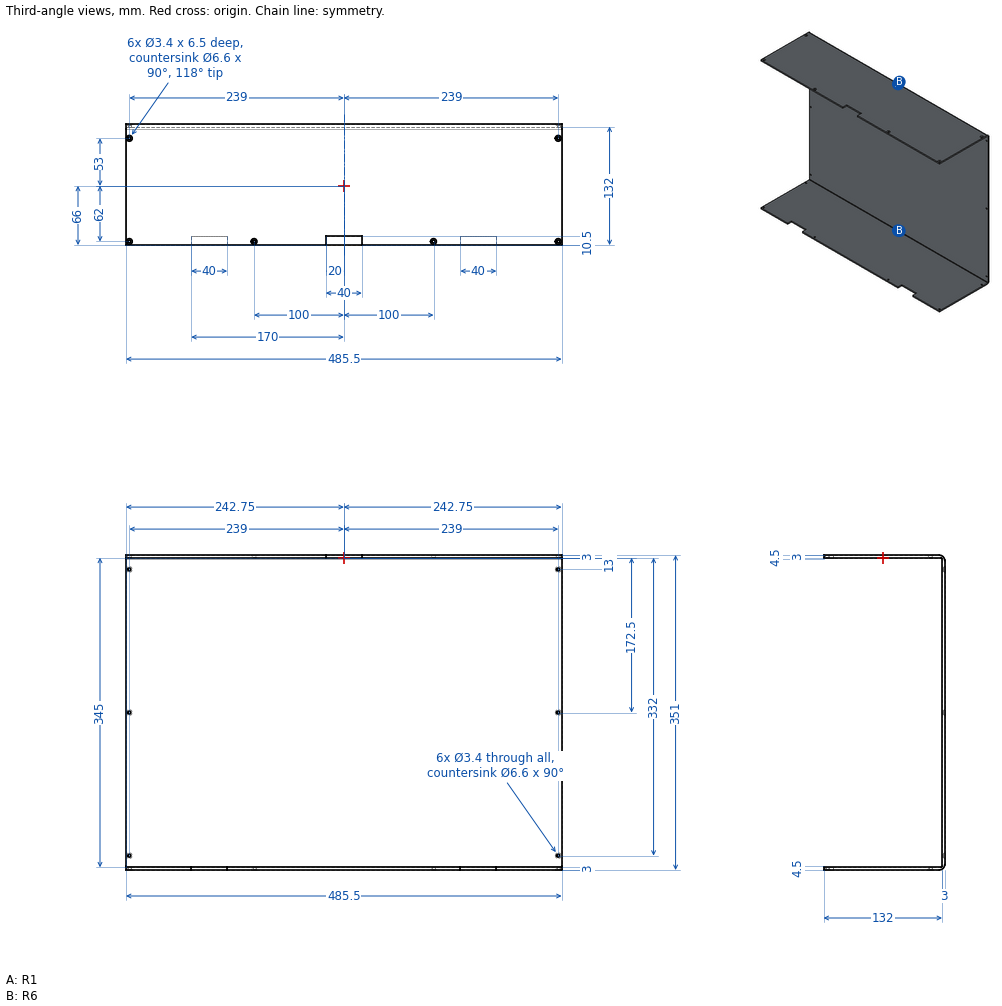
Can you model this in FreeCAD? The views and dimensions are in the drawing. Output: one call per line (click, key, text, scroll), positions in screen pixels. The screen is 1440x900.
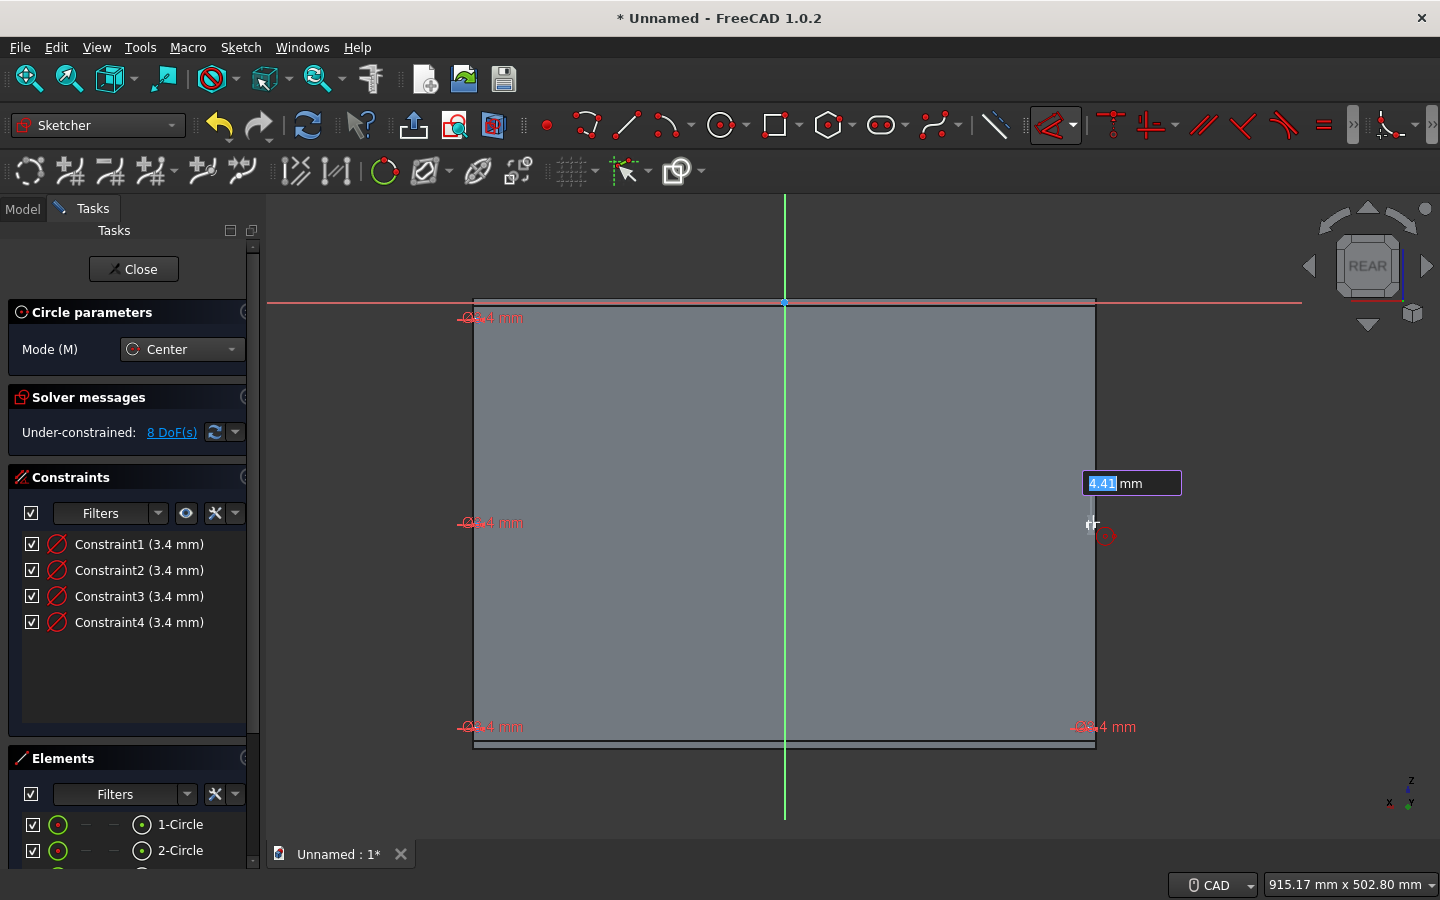
text(3.4)
key(Return)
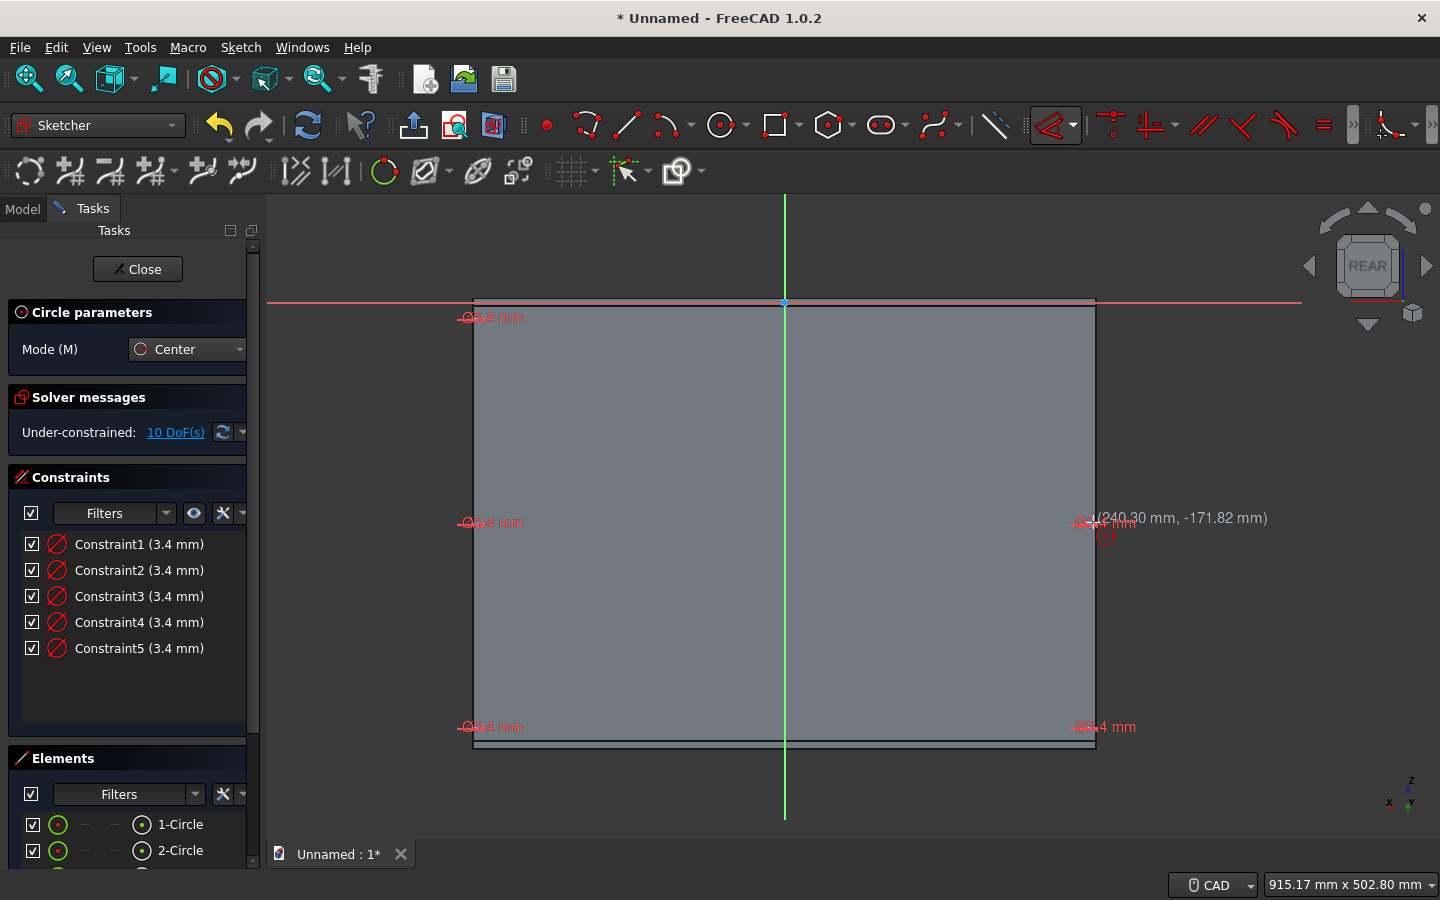
scroll(1091, 319, up, 12)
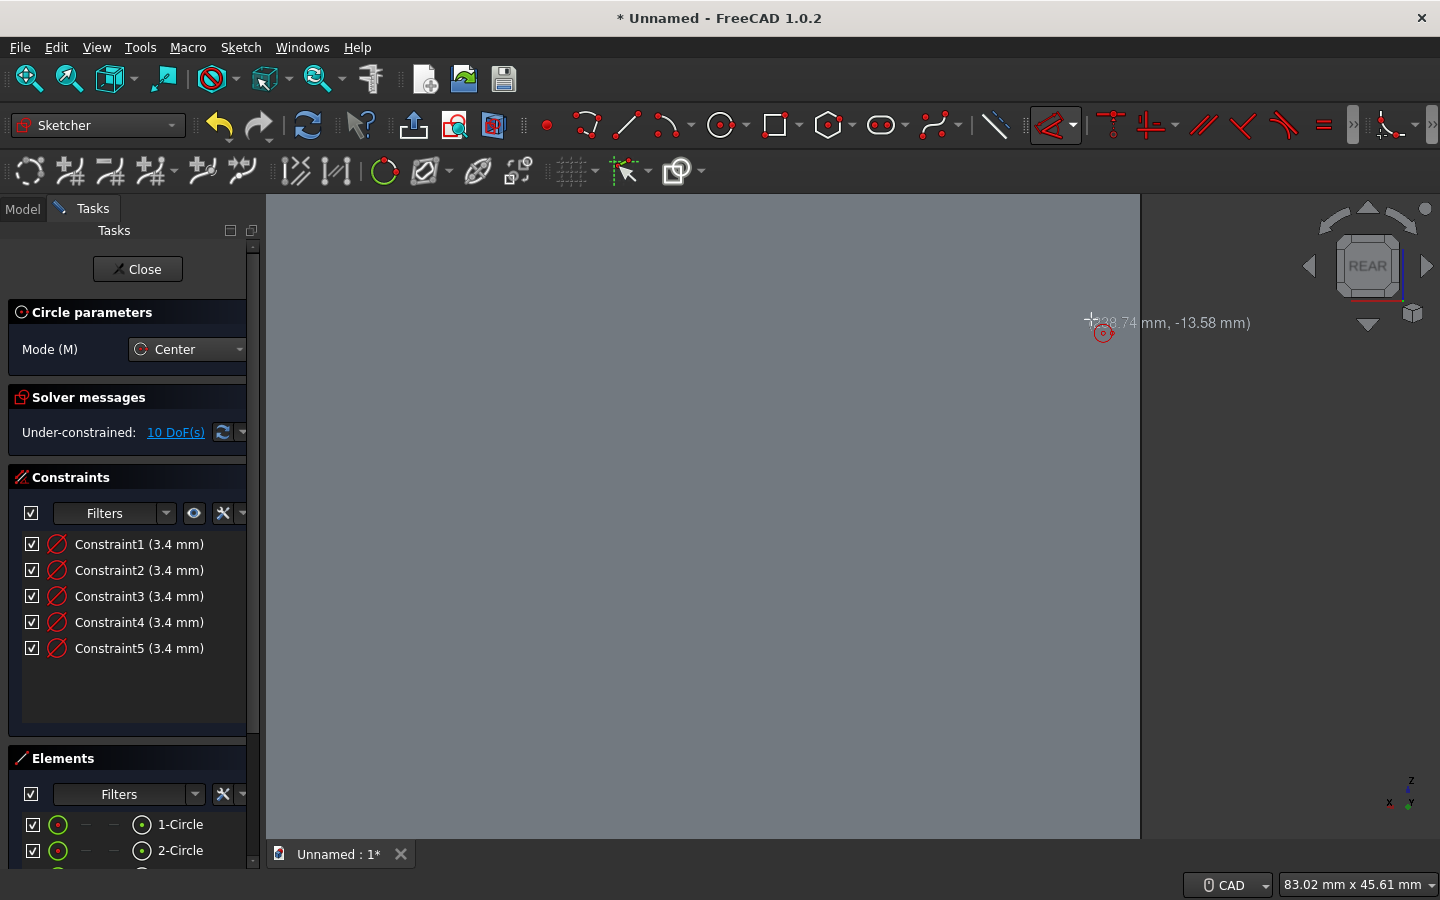
scroll(1091, 319, down, 12)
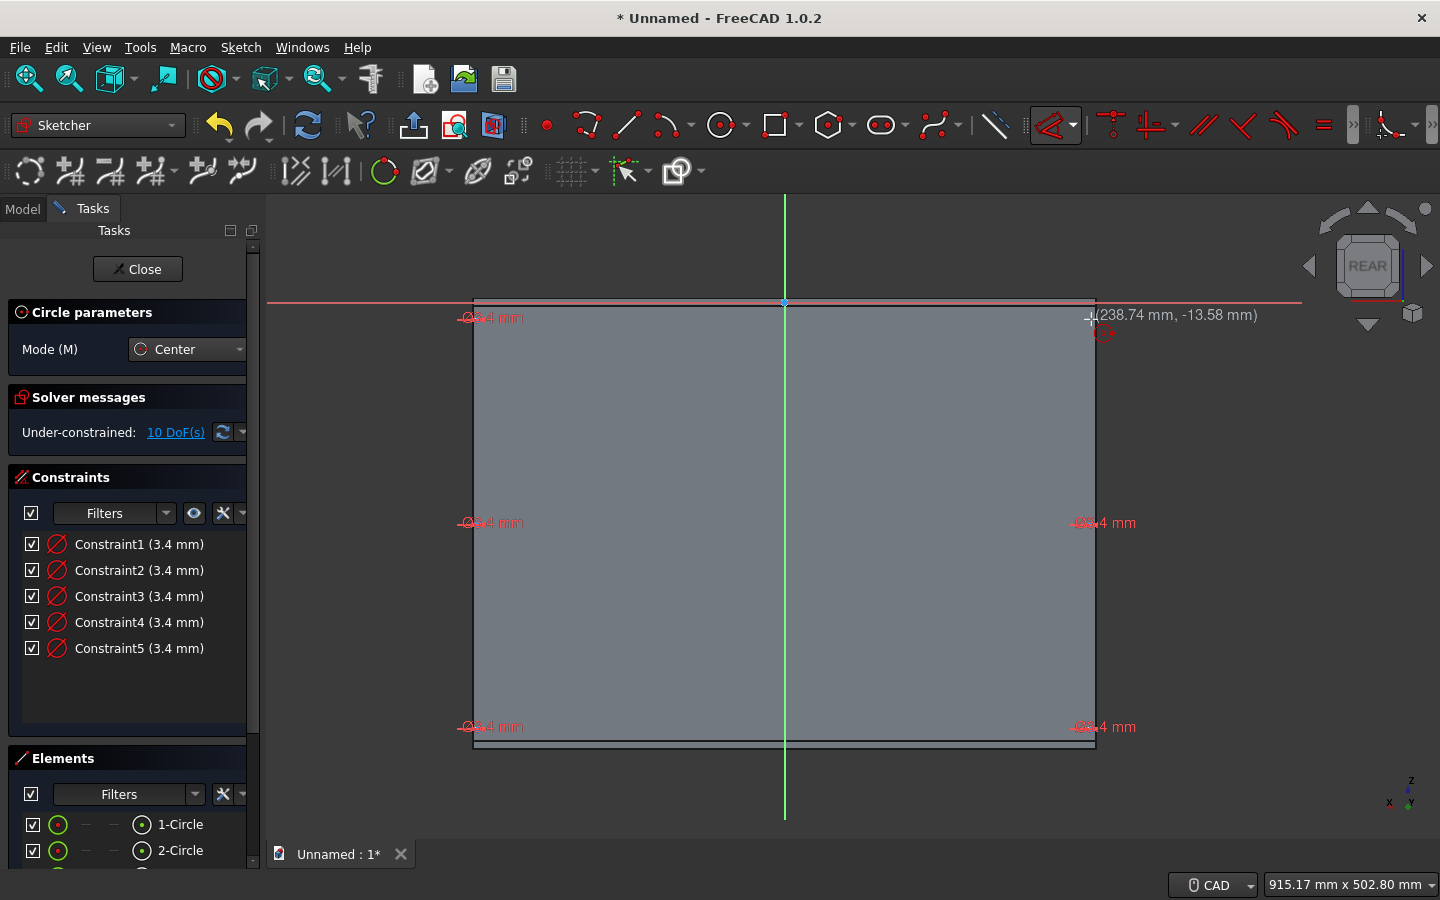
click(1091, 319)
move(1093, 318)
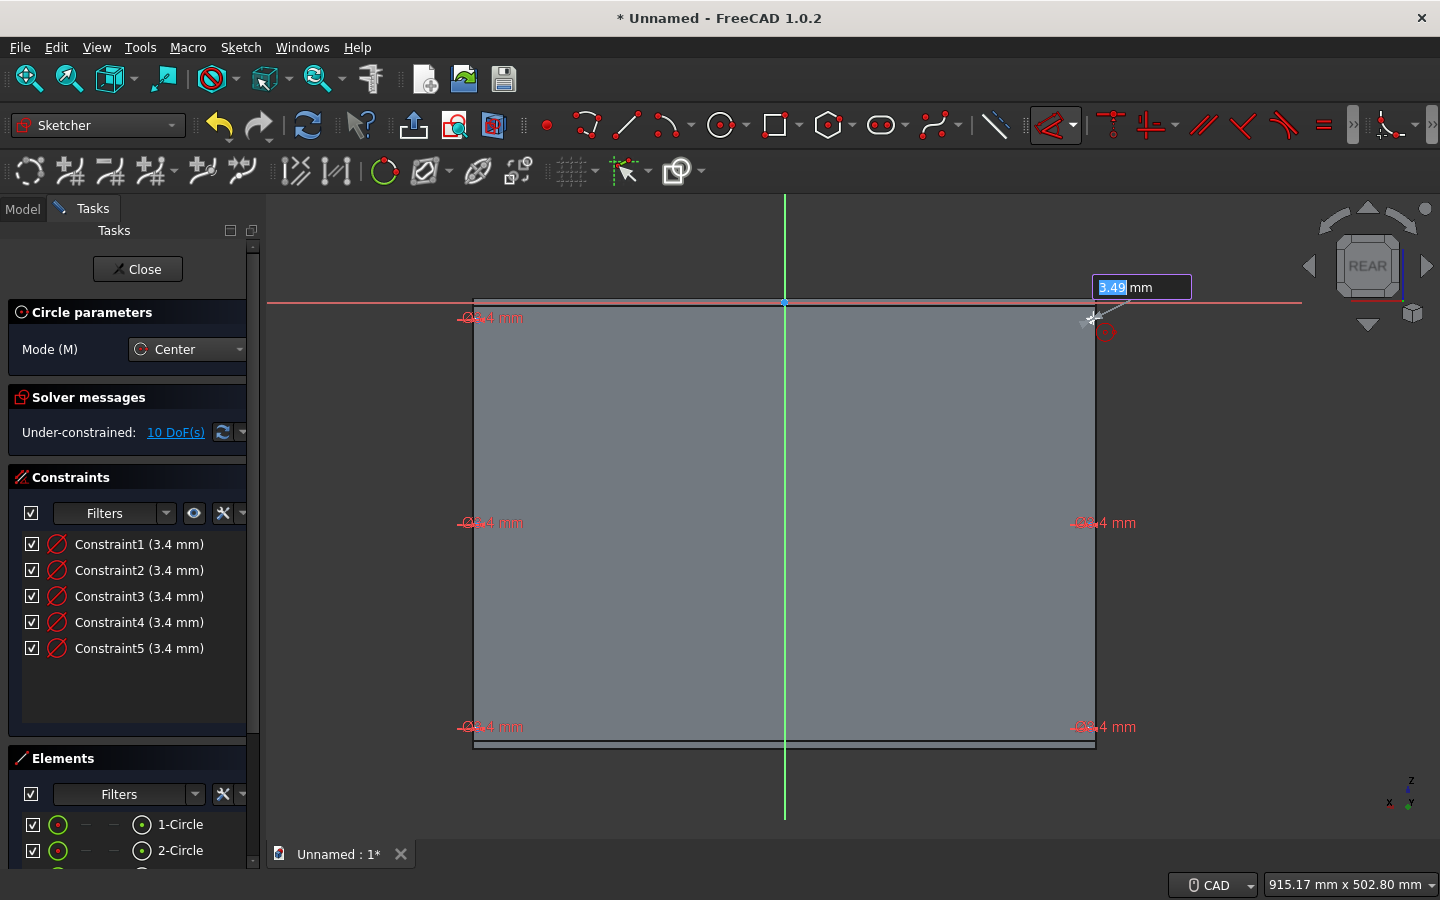
text(3.4)
key(Return)
key(Escape)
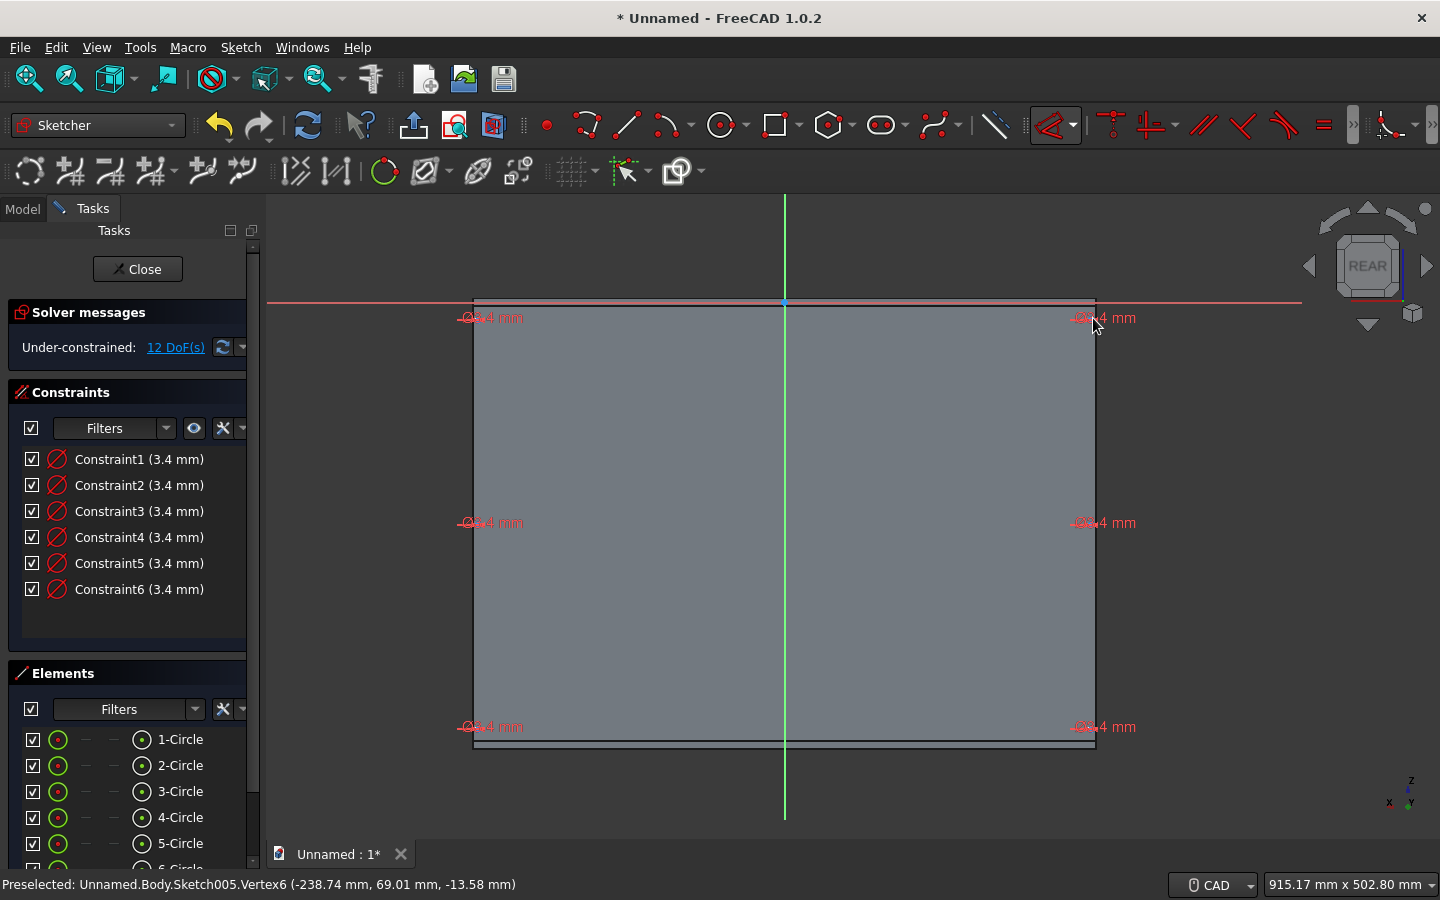
click(478, 729)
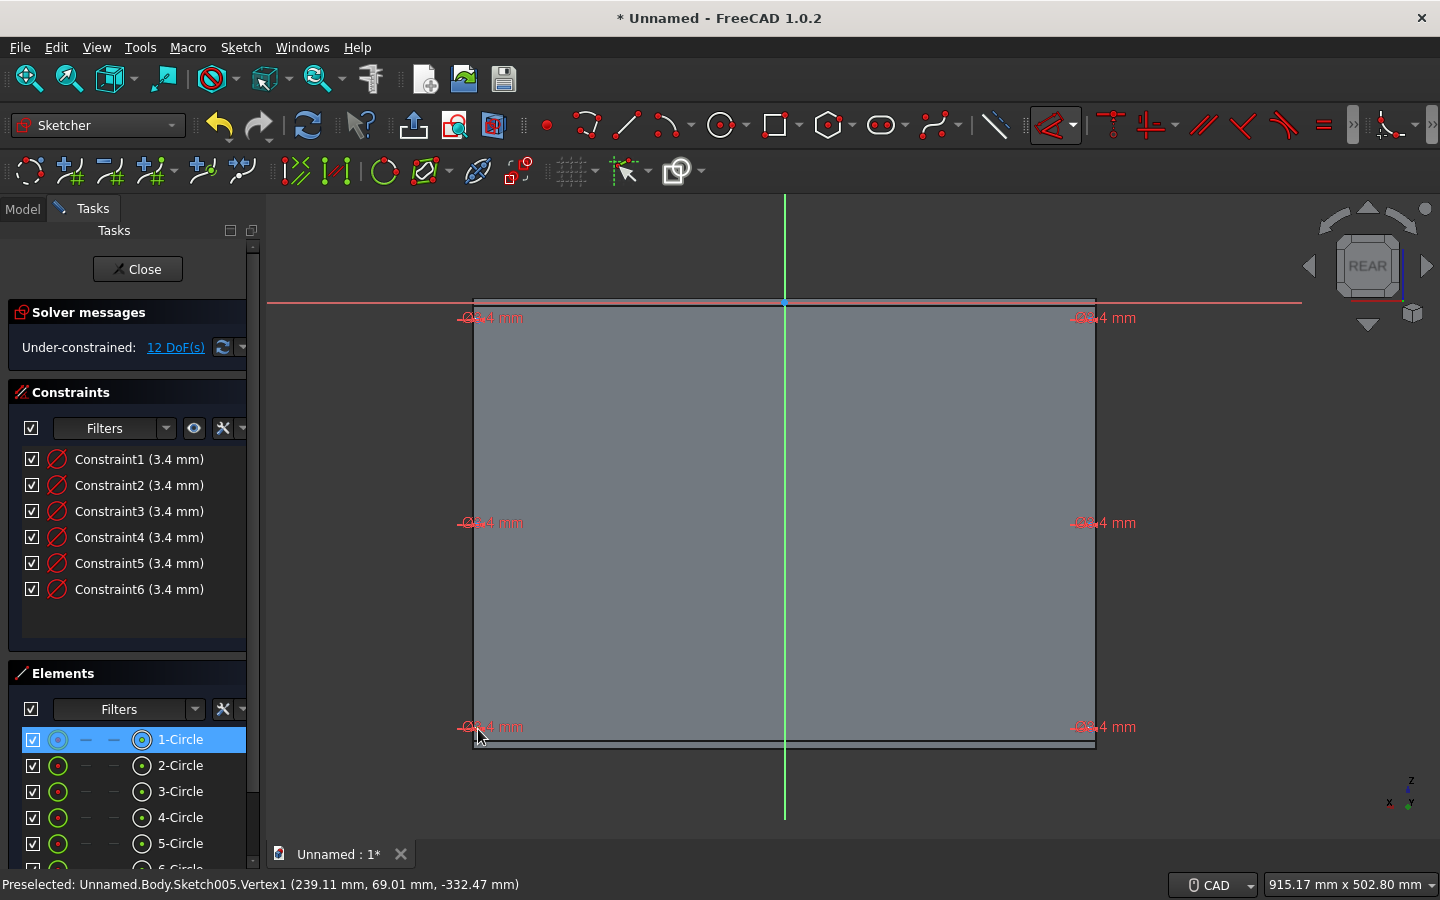
click(478, 525)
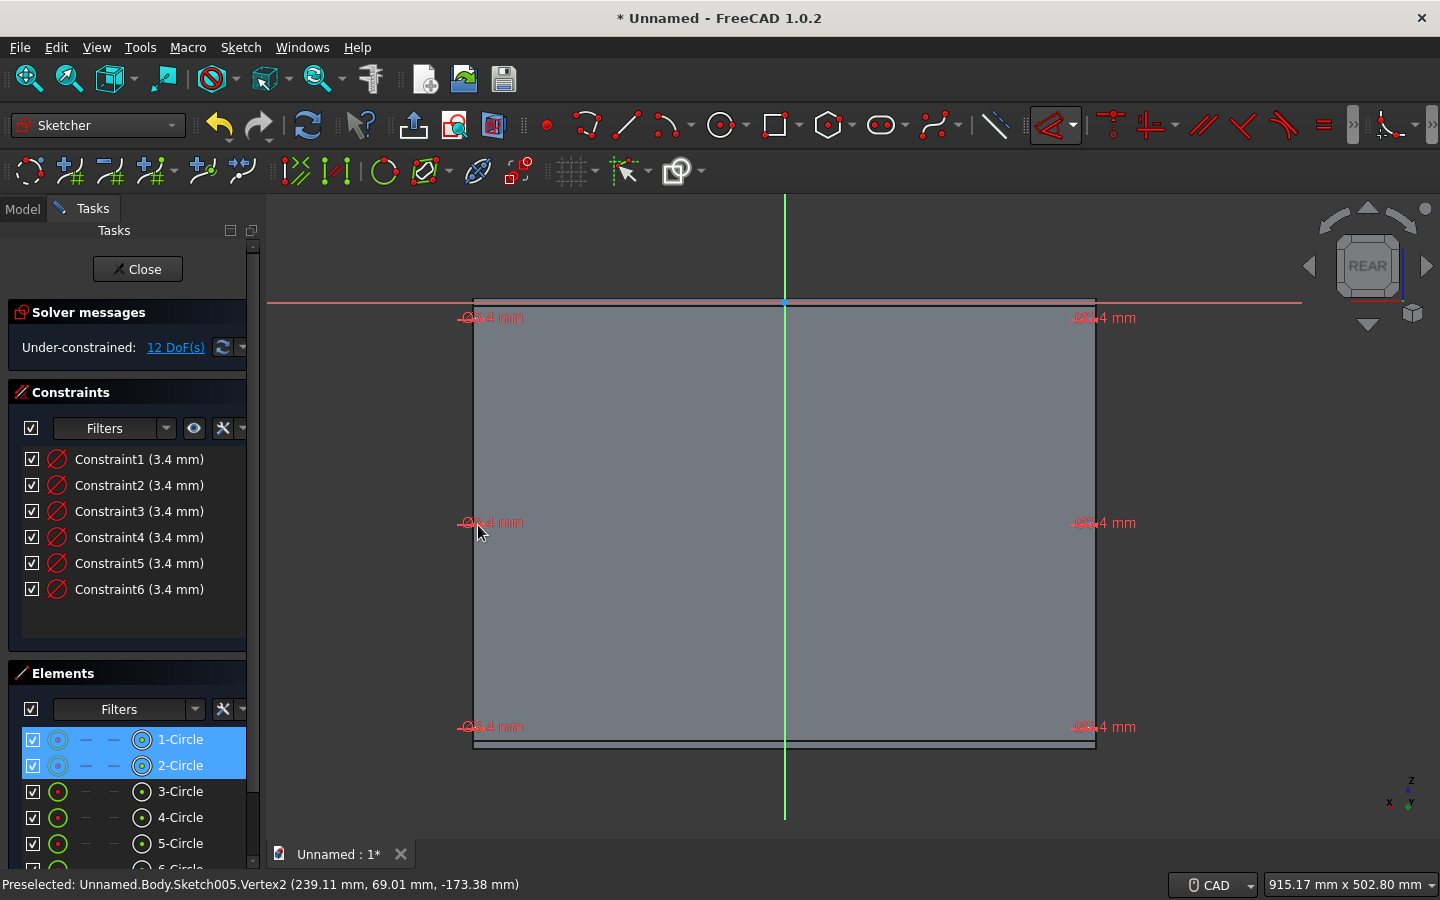
click(1178, 126)